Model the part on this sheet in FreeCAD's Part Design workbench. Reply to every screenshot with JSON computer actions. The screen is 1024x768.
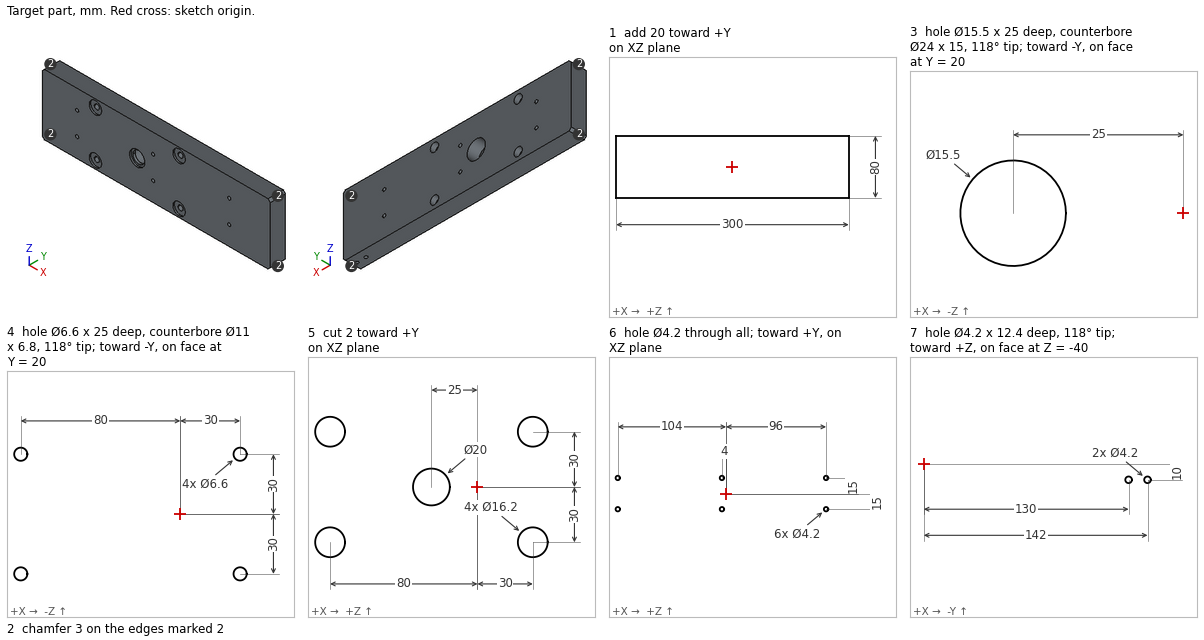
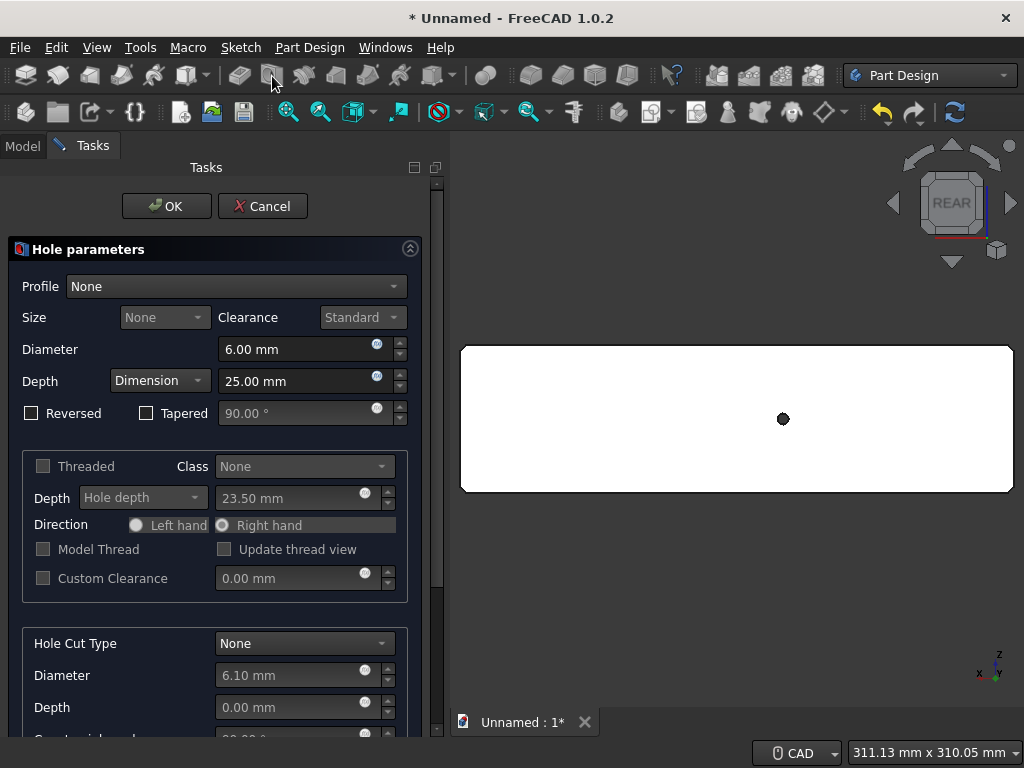
{"action": "triple_click", "coordinate": [305, 349]}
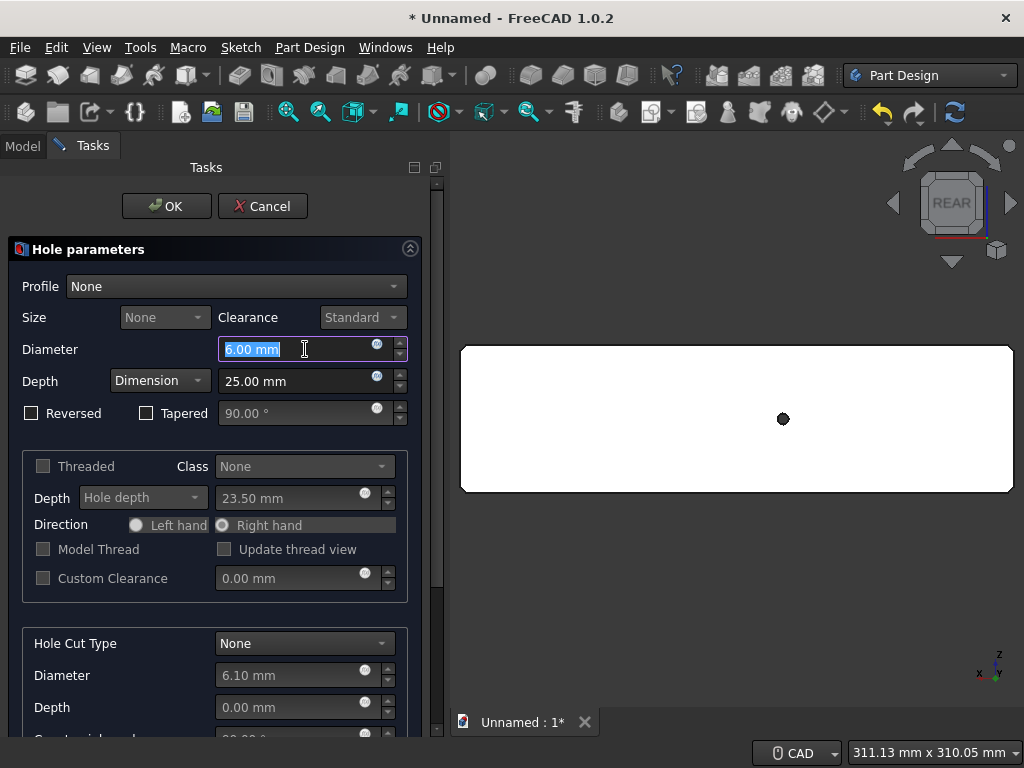
{"action": "type", "text": "15.5"}
{"action": "key", "text": "Tab"}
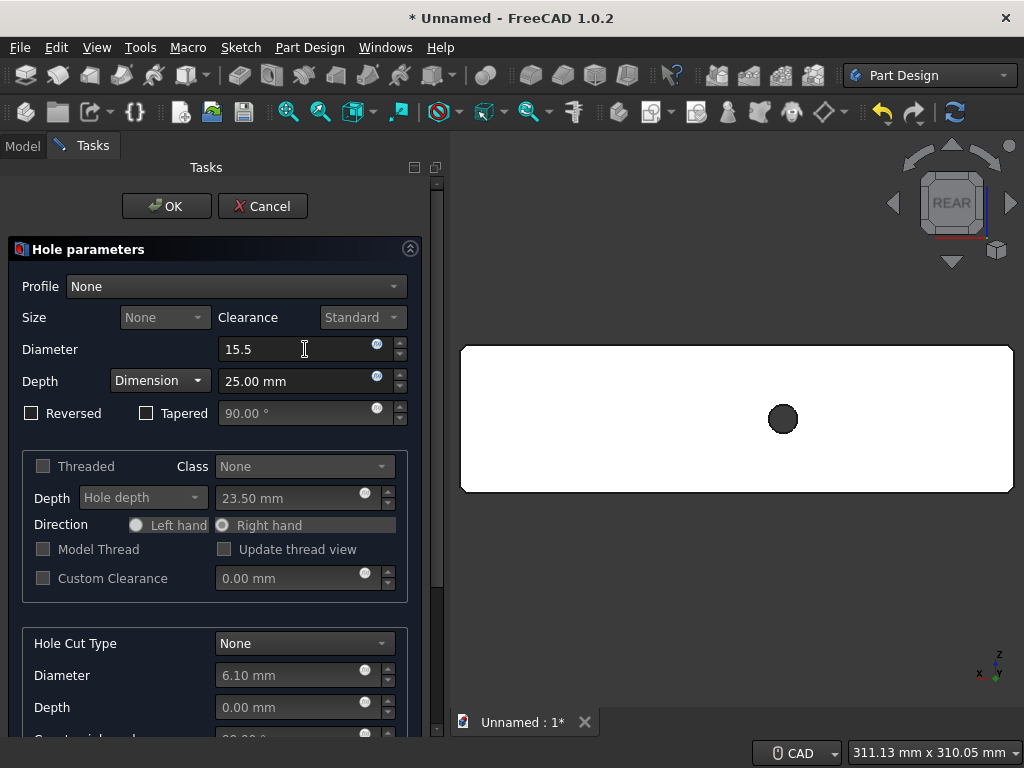
{"action": "triple_click", "coordinate": [305, 381]}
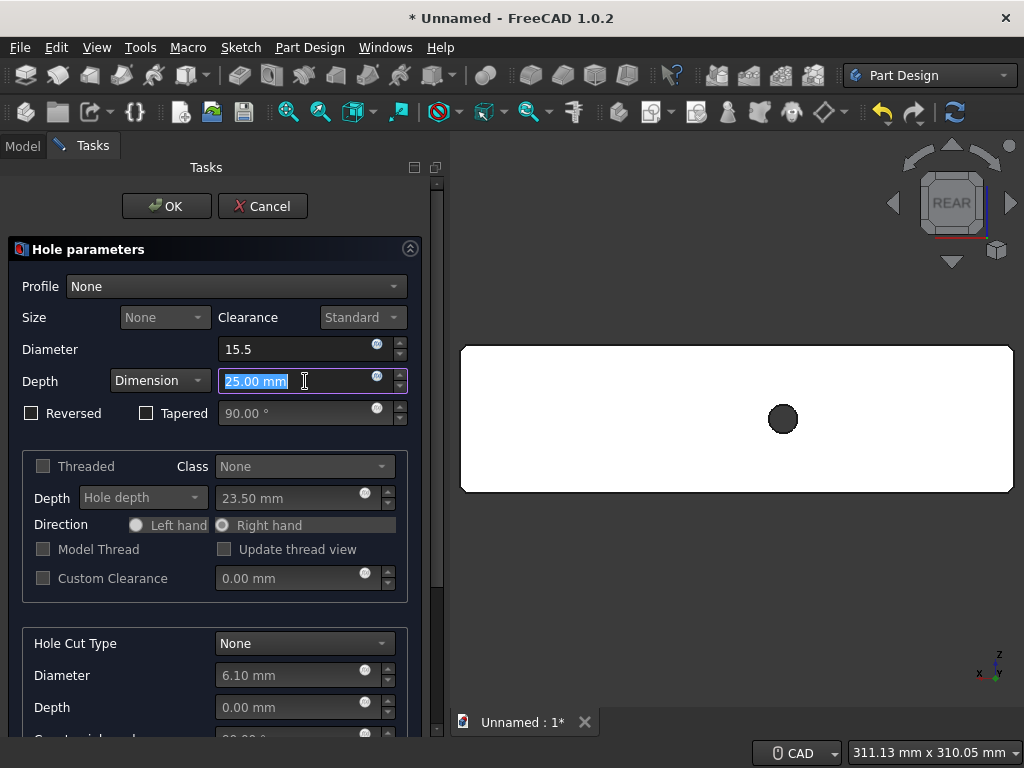
{"action": "type", "text": "25"}
{"action": "key", "text": "Tab"}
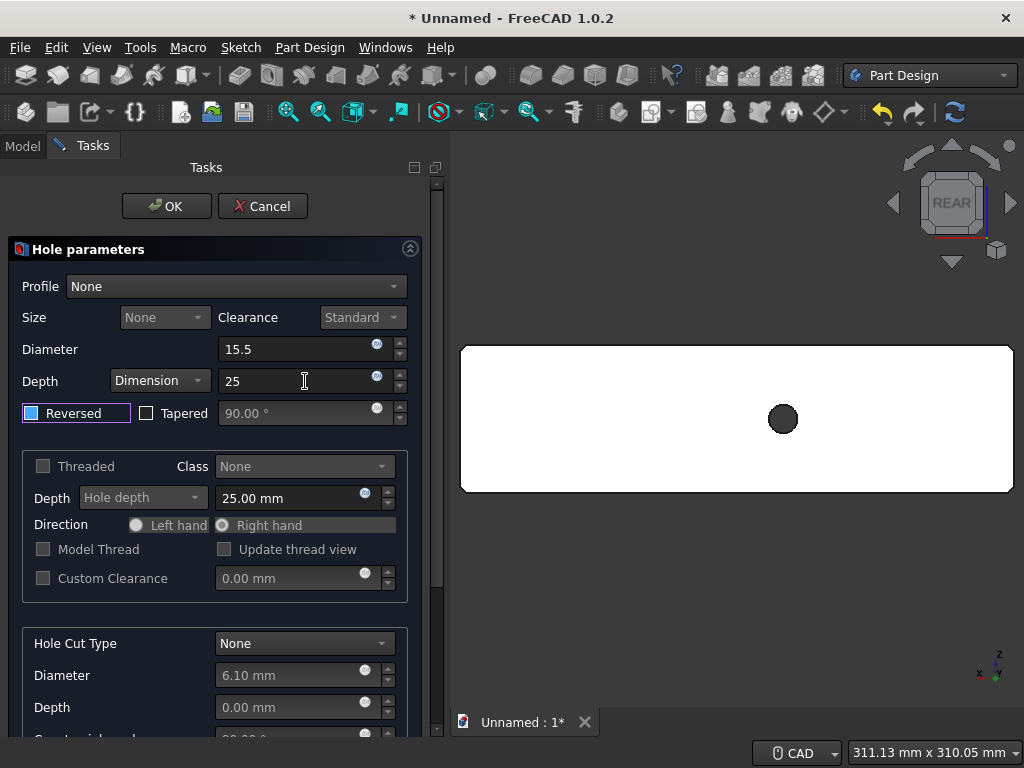
{"action": "left_click", "coordinate": [306, 644]}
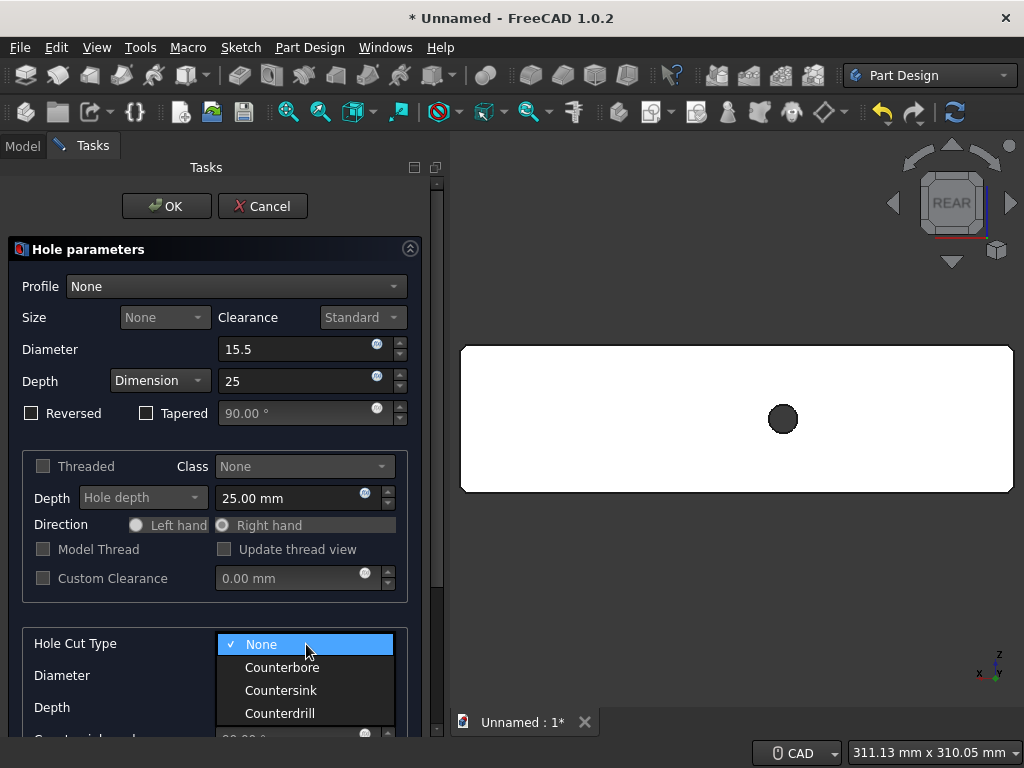
{"action": "left_click", "coordinate": [304, 668]}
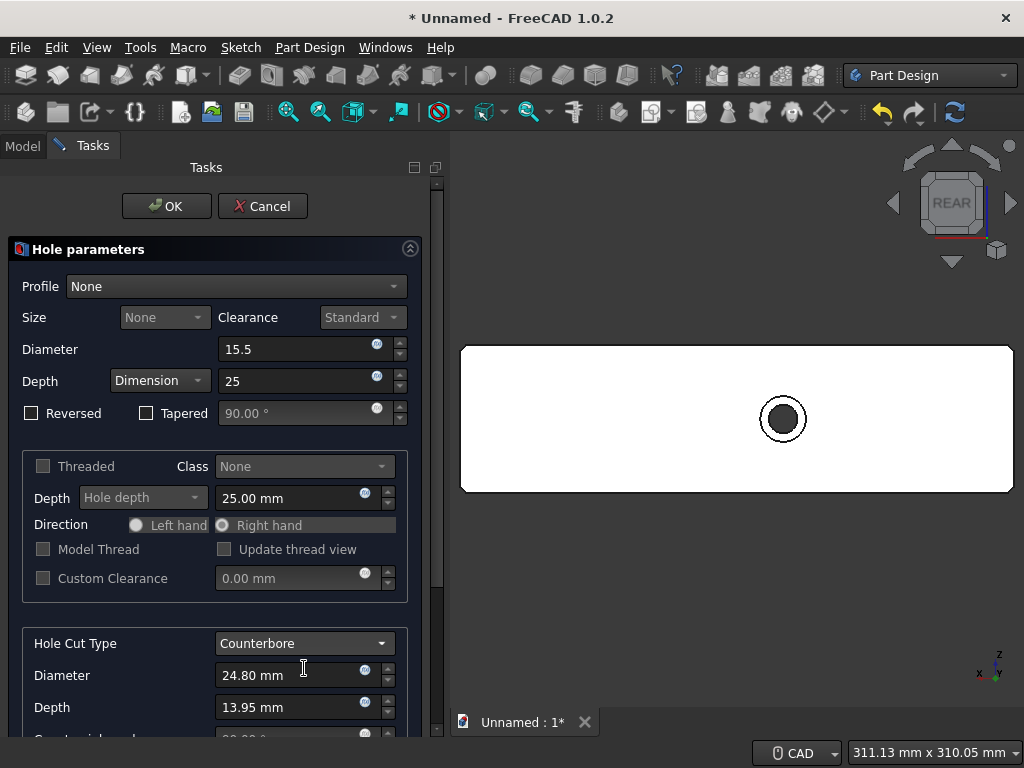
{"action": "triple_click", "coordinate": [298, 675]}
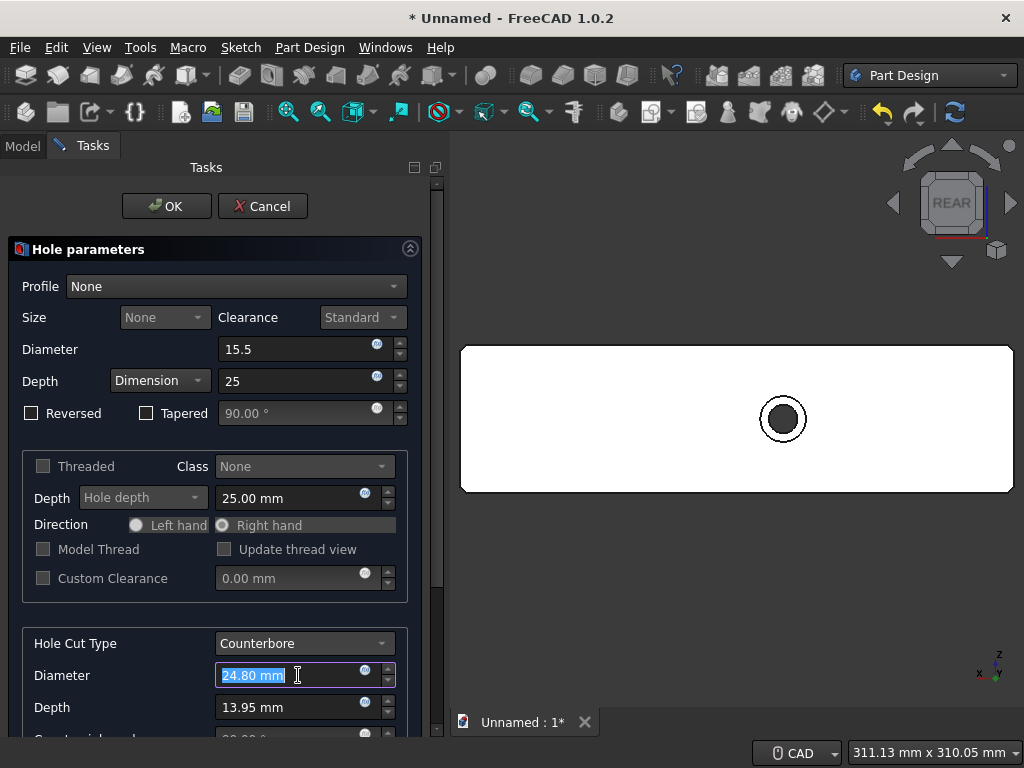
{"action": "type", "text": "24"}
{"action": "key", "text": "Tab"}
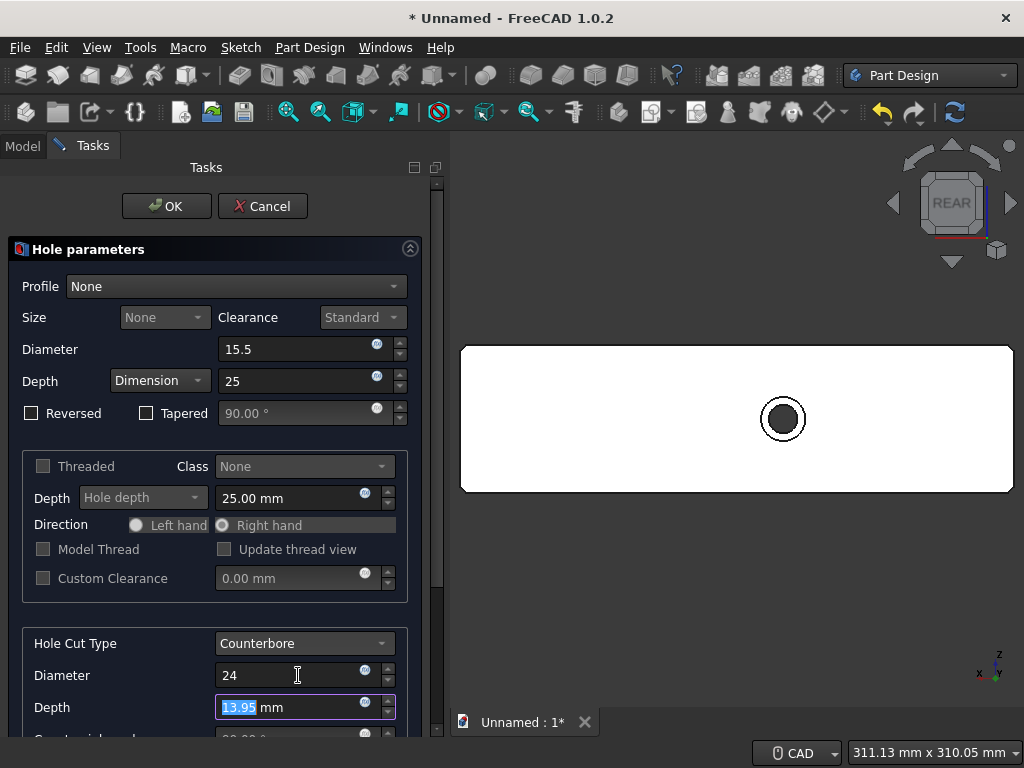
{"action": "type", "text": "15"}
{"action": "key", "text": "Tab"}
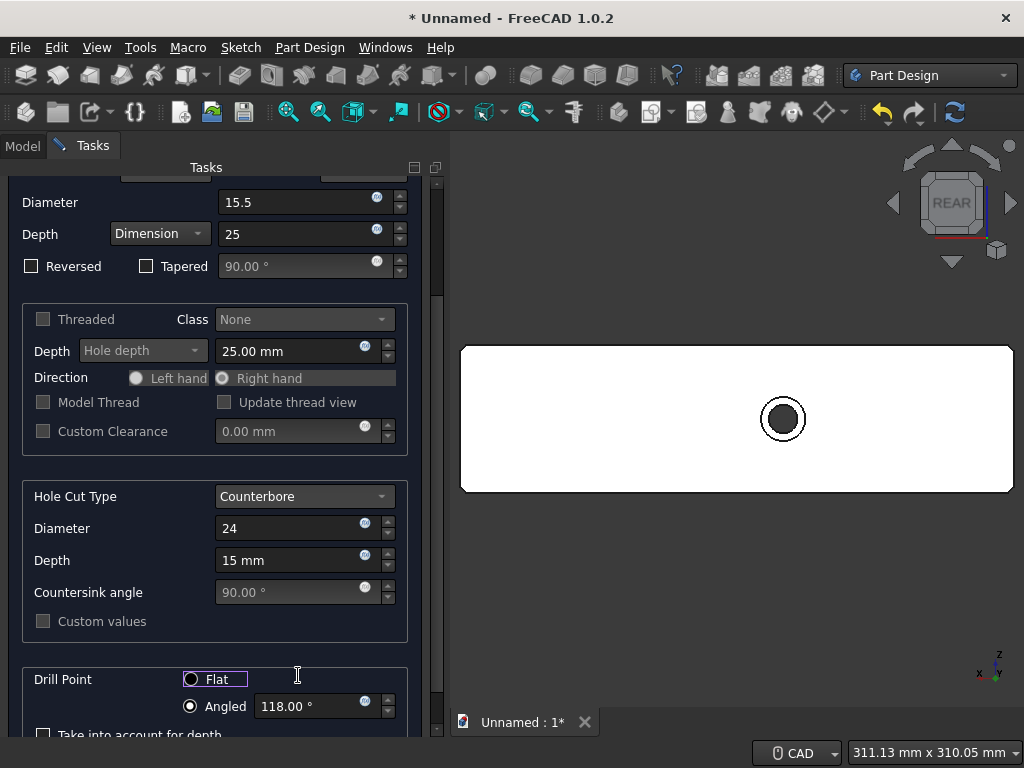
{"action": "scroll", "coordinate": [437, 456], "scroll_direction": "up", "scroll_amount": 4}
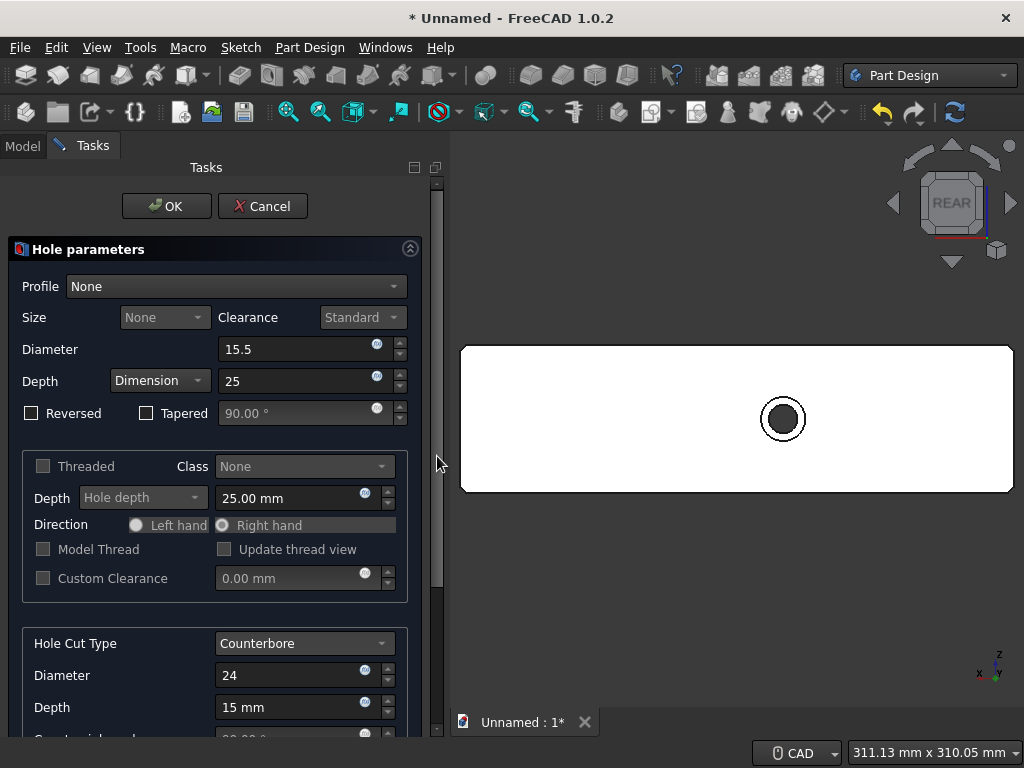
{"action": "left_click", "coordinate": [167, 206]}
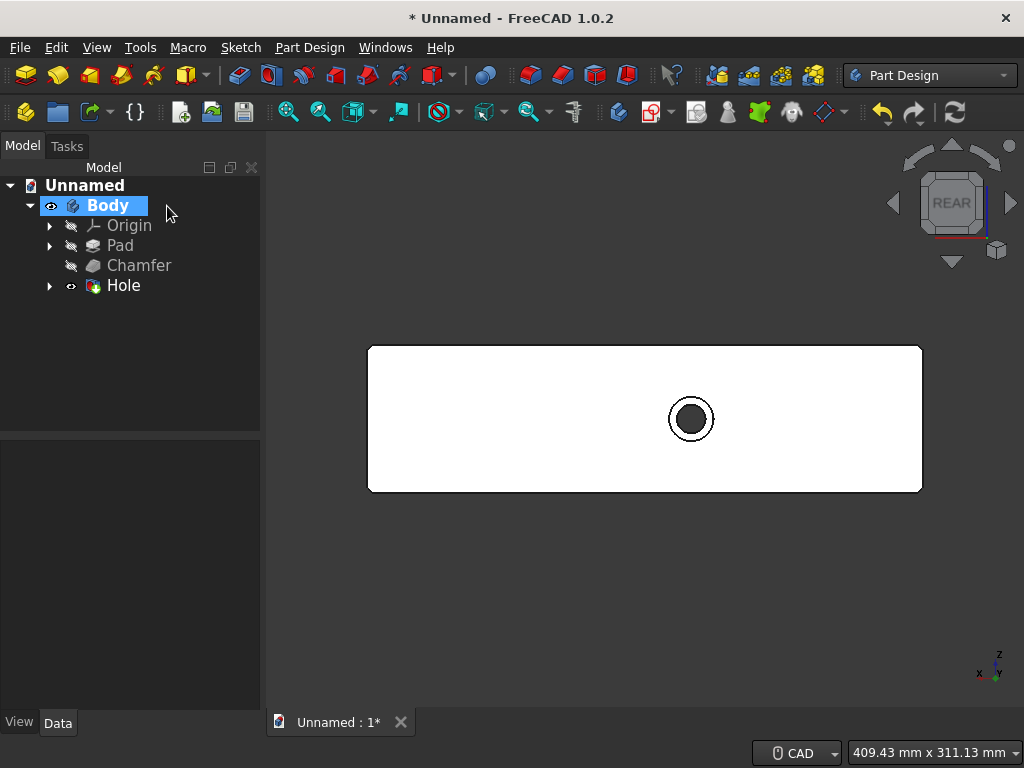
{"action": "left_click", "coordinate": [486, 418]}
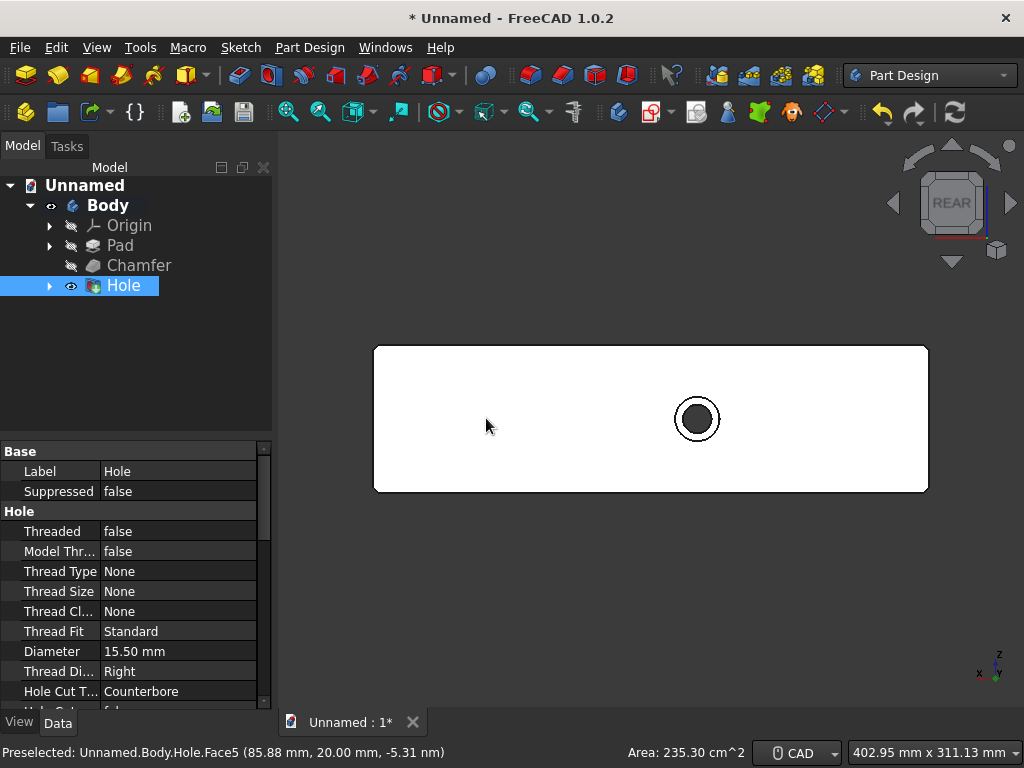
{"action": "left_click", "coordinate": [652, 112]}